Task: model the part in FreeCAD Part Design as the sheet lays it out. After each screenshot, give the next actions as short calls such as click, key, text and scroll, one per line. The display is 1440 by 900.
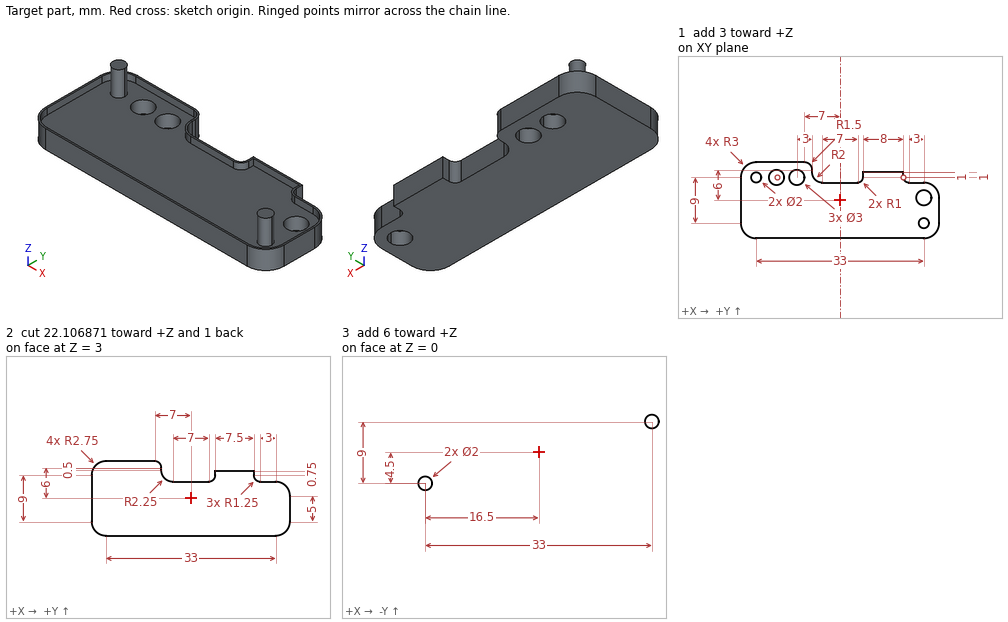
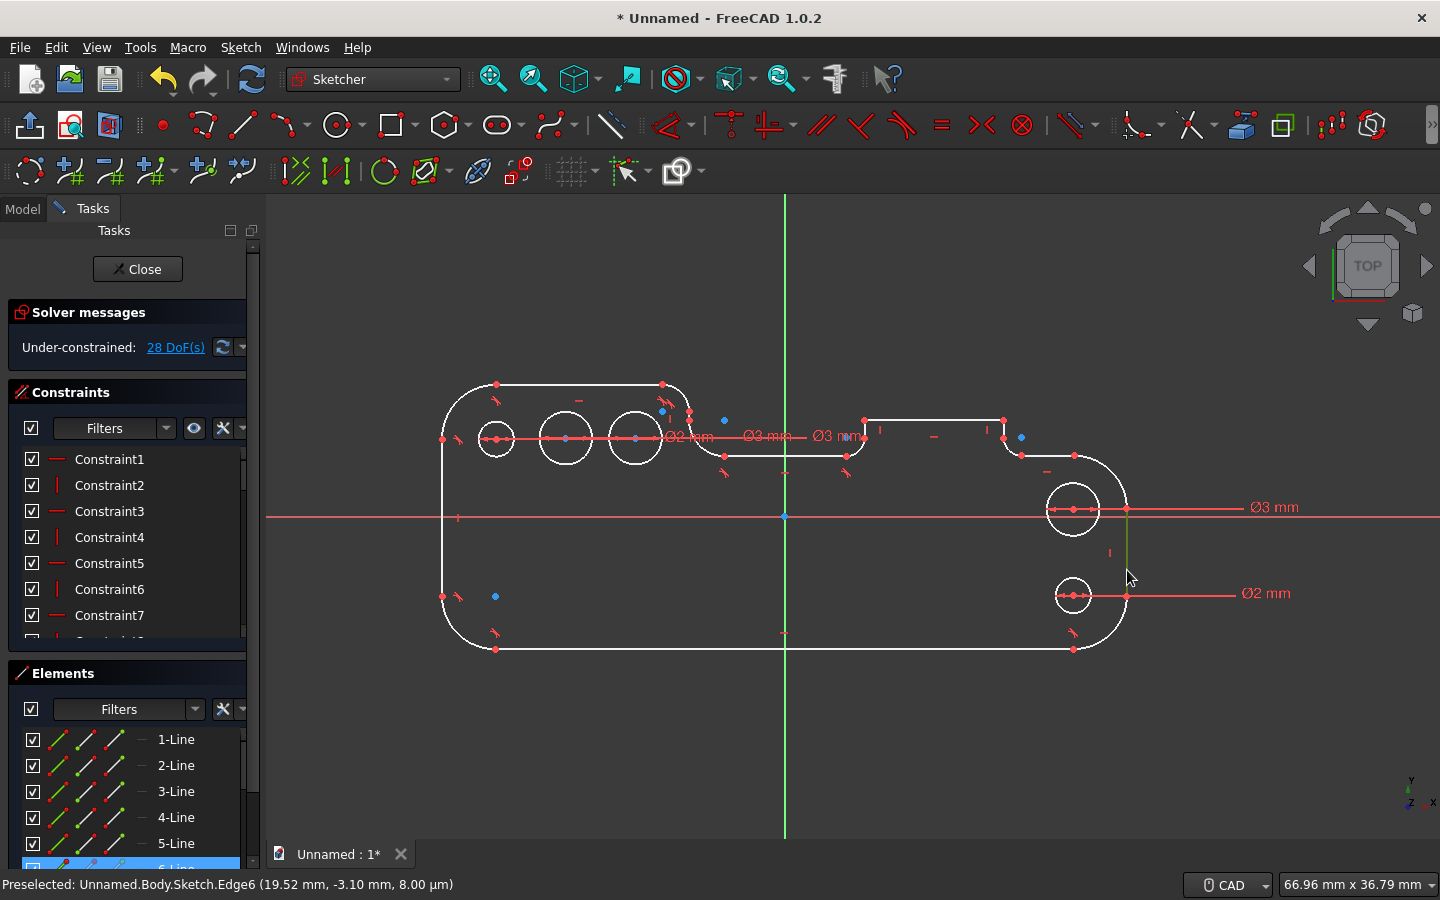
click(1098, 643)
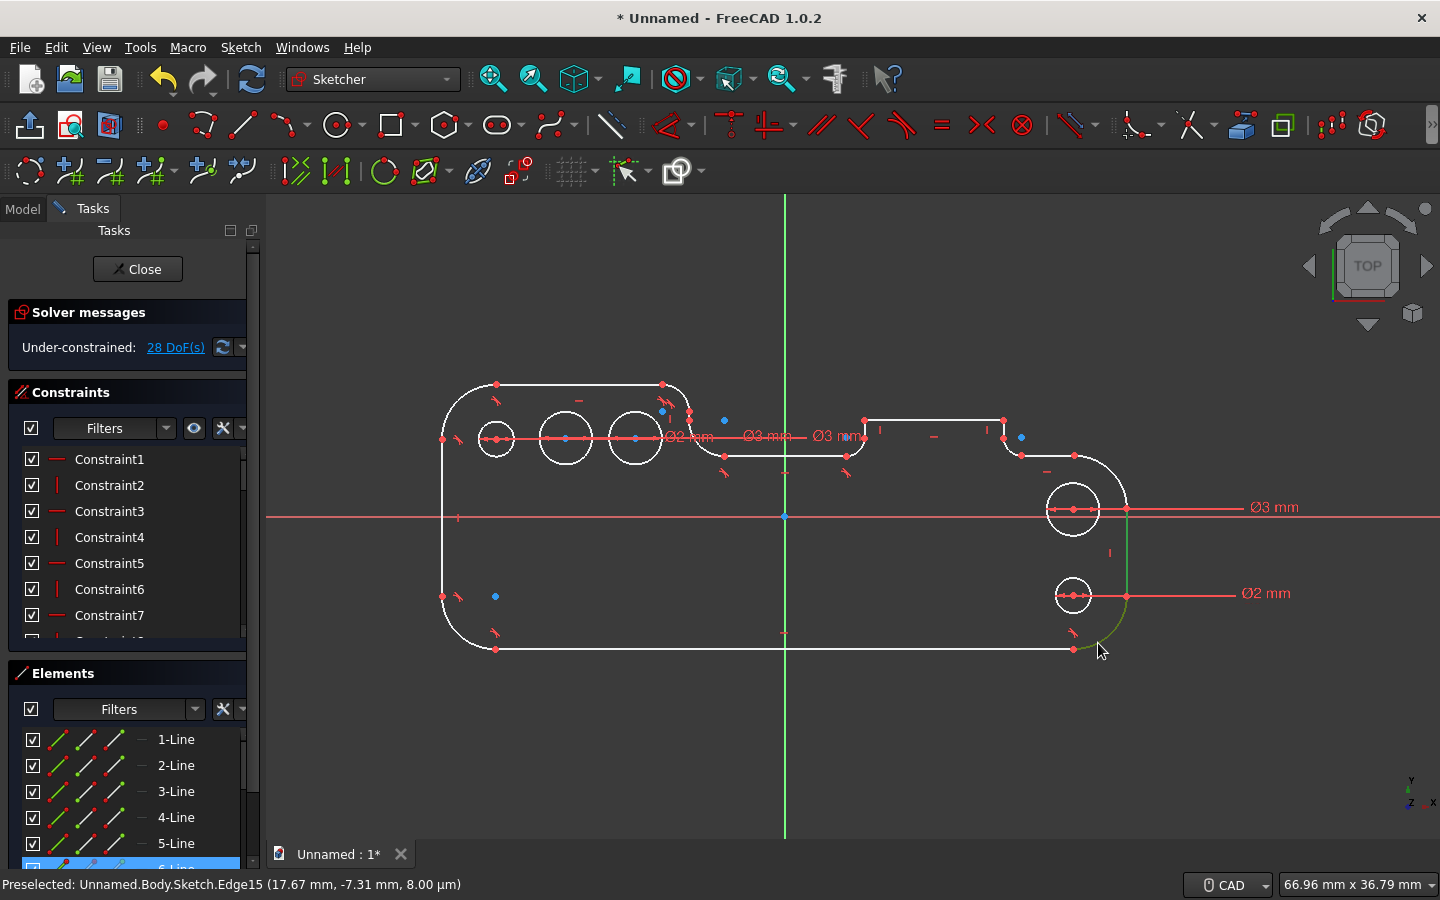
click(902, 126)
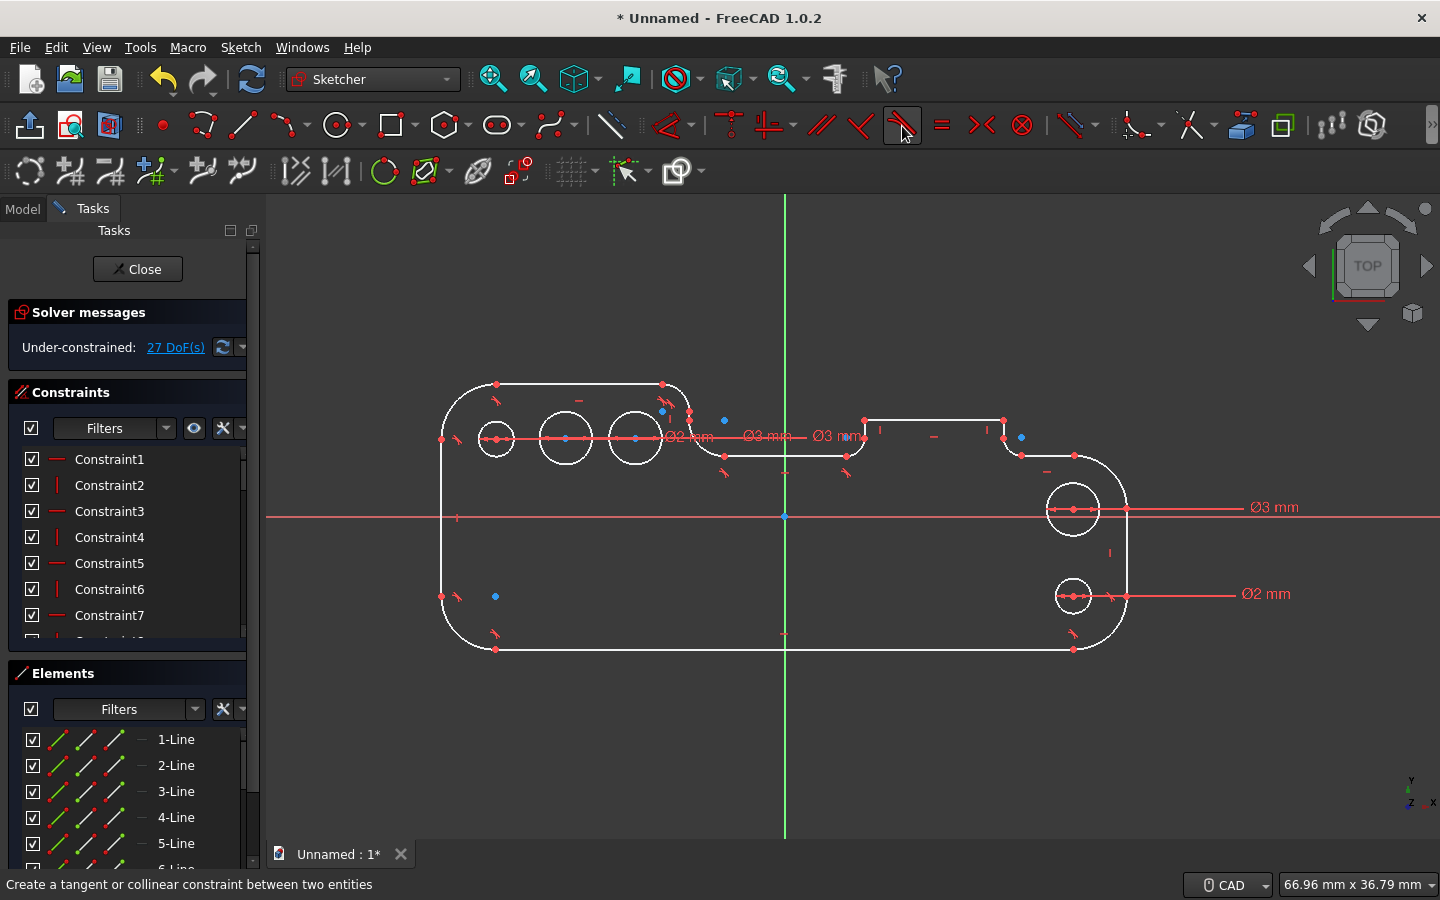
click(1127, 570)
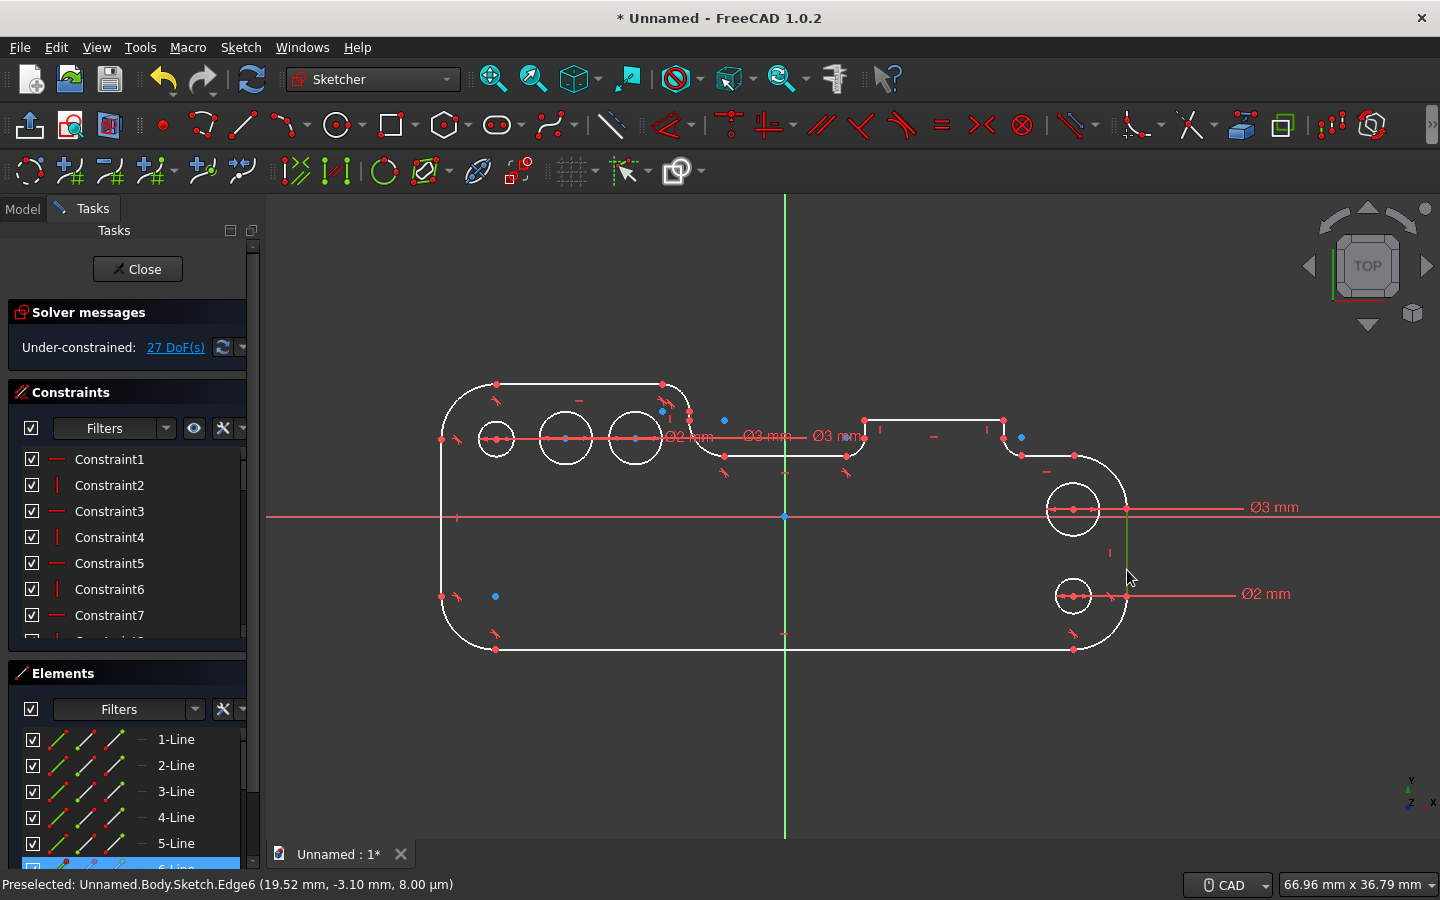
click(1121, 485)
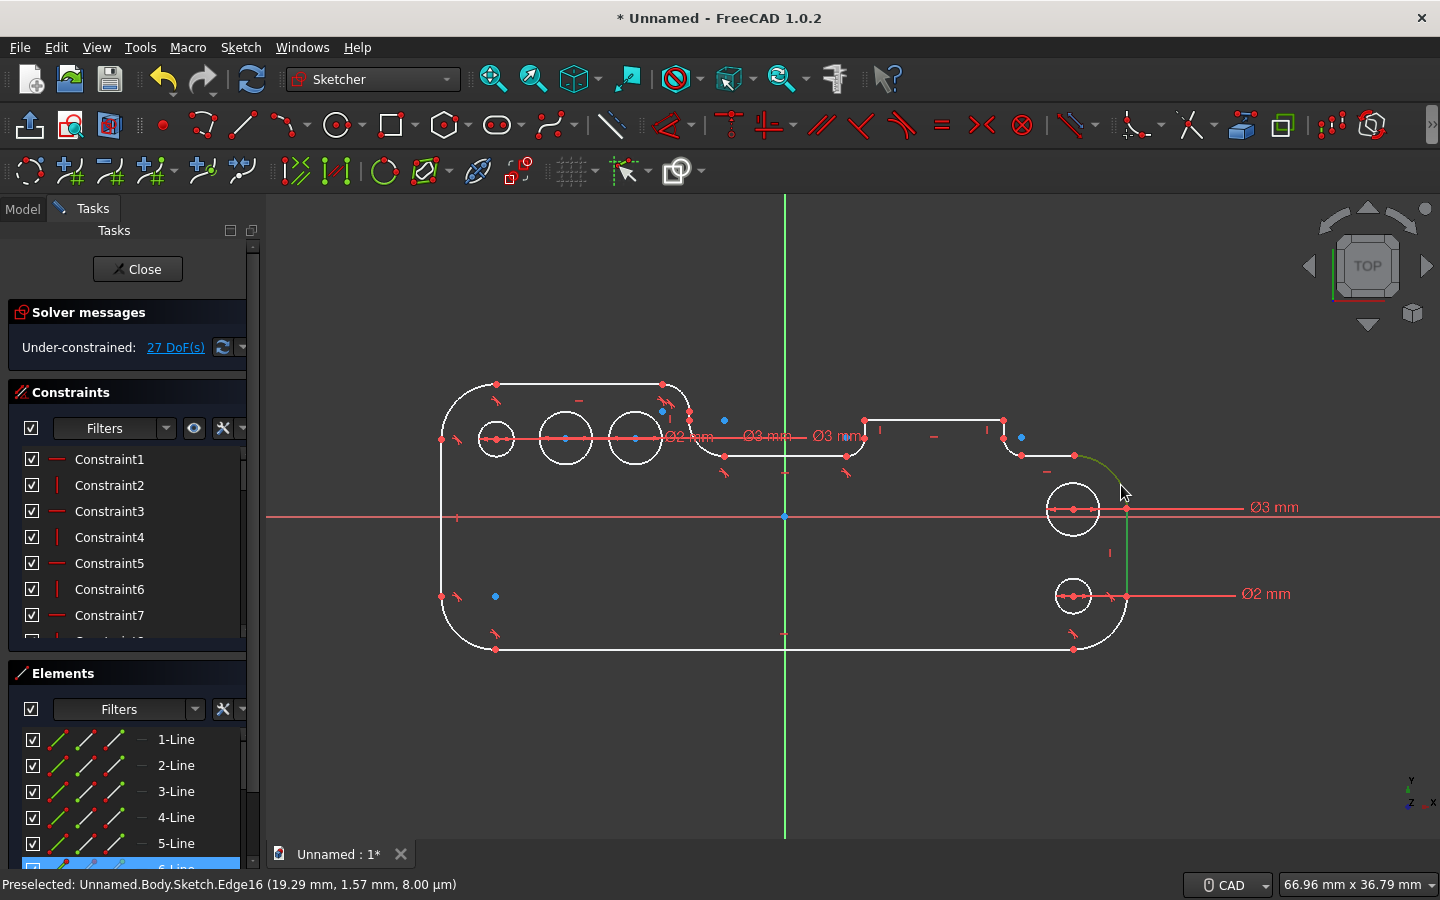
click(902, 126)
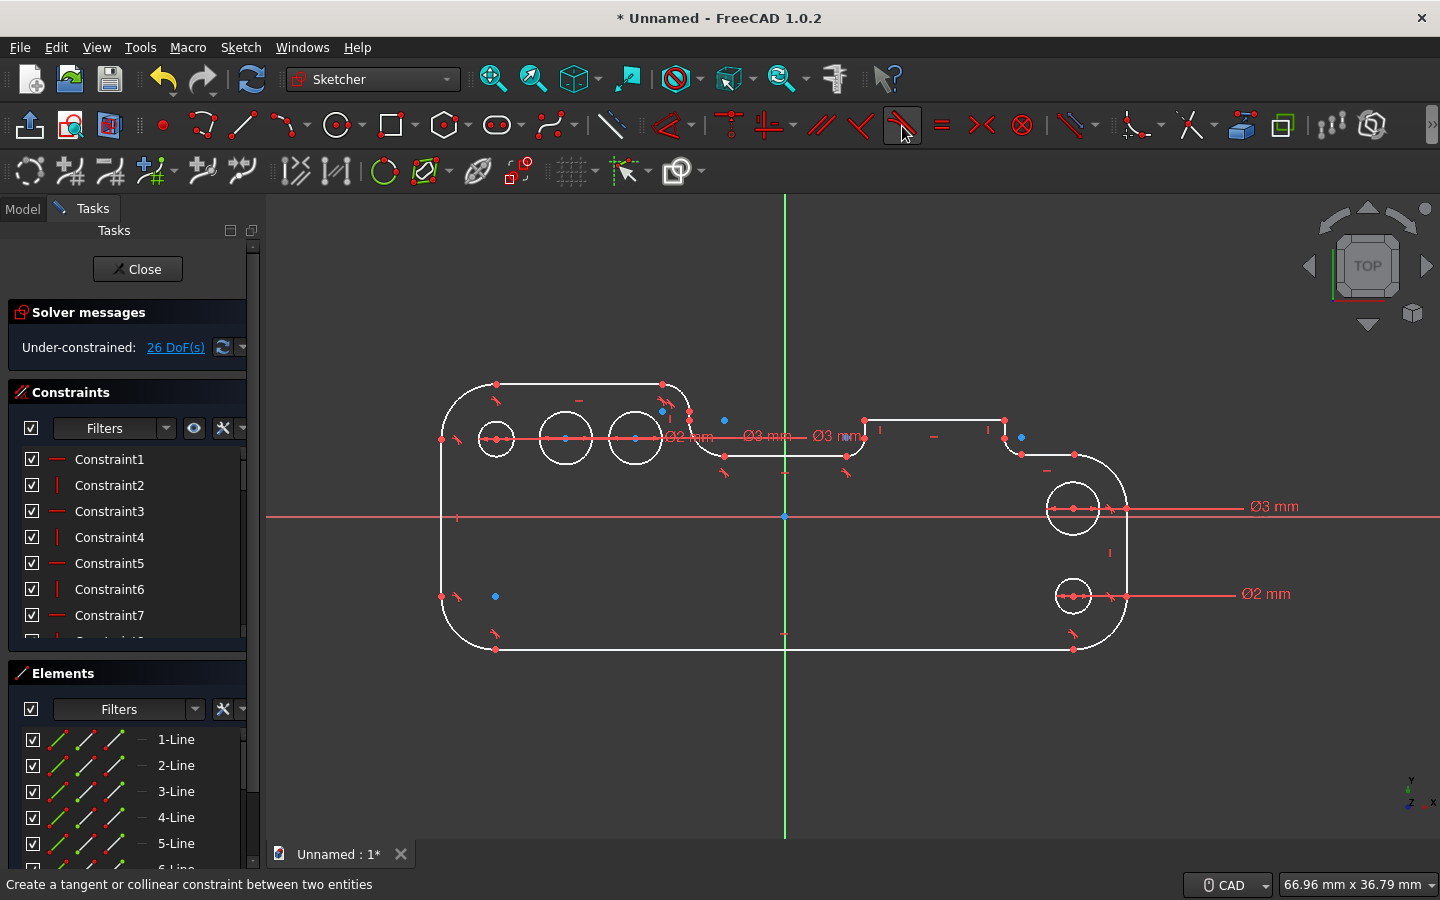
click(1058, 455)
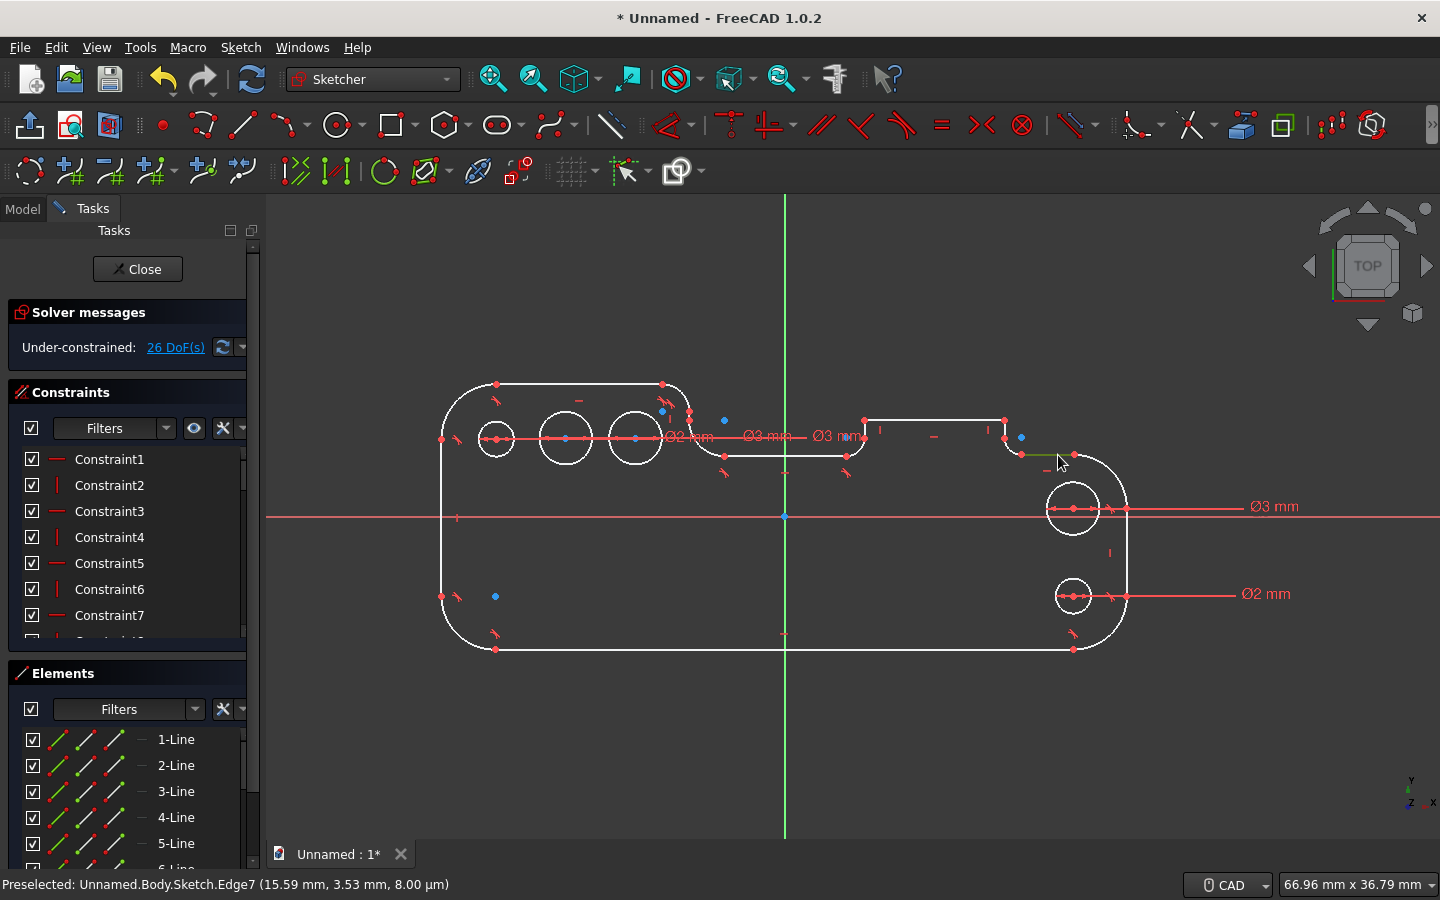
click(1121, 484)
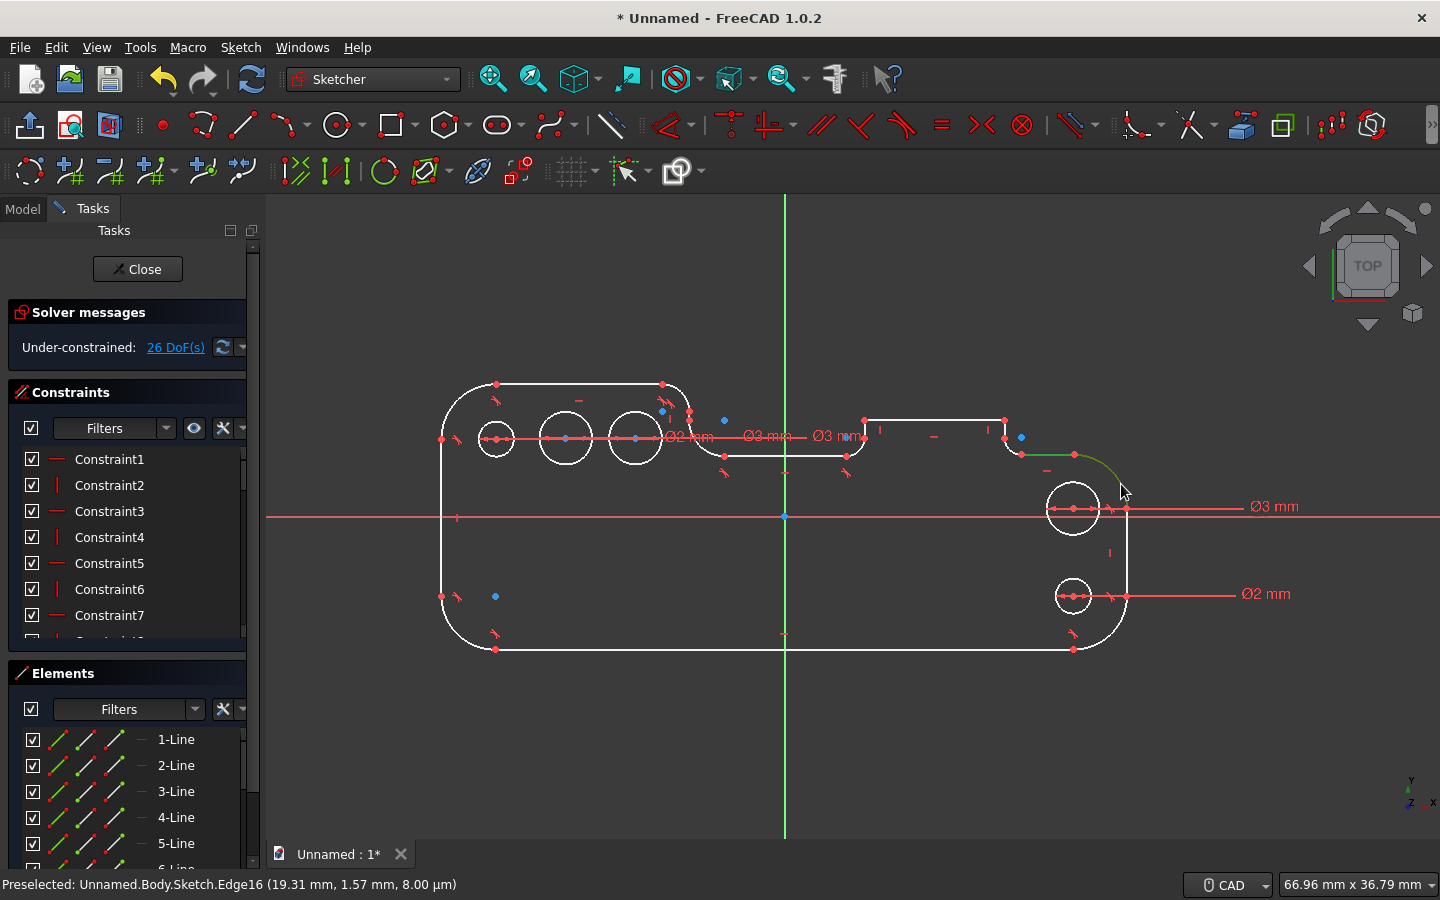
click(902, 126)